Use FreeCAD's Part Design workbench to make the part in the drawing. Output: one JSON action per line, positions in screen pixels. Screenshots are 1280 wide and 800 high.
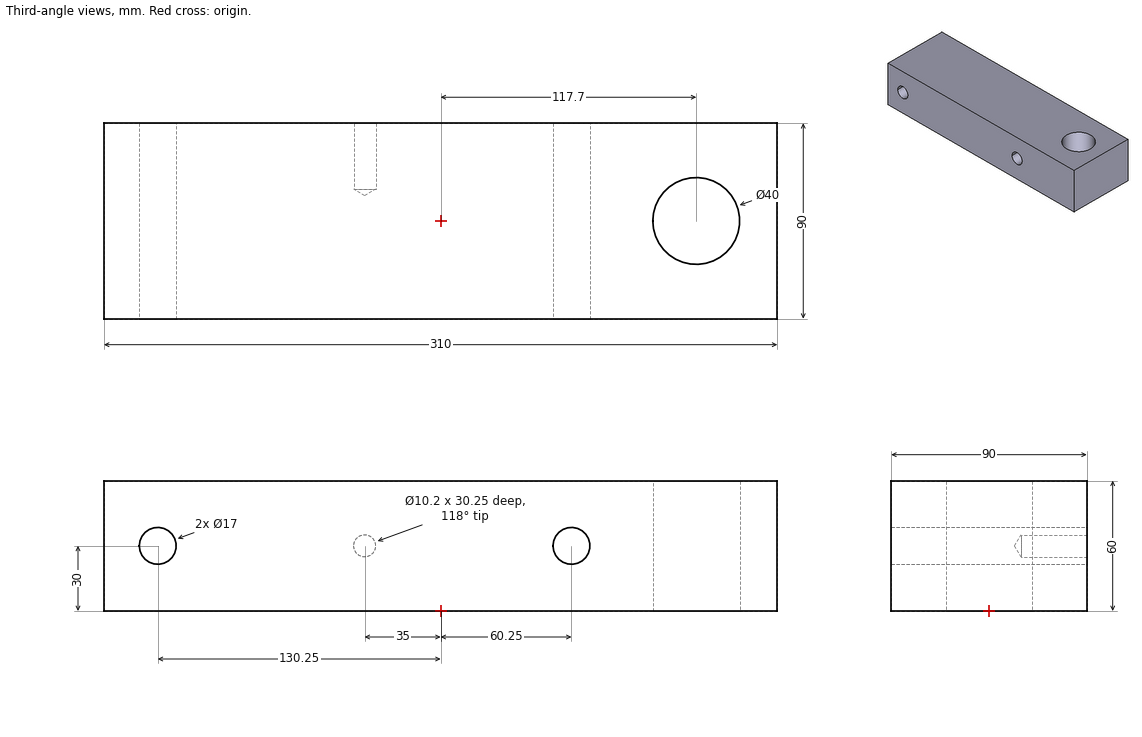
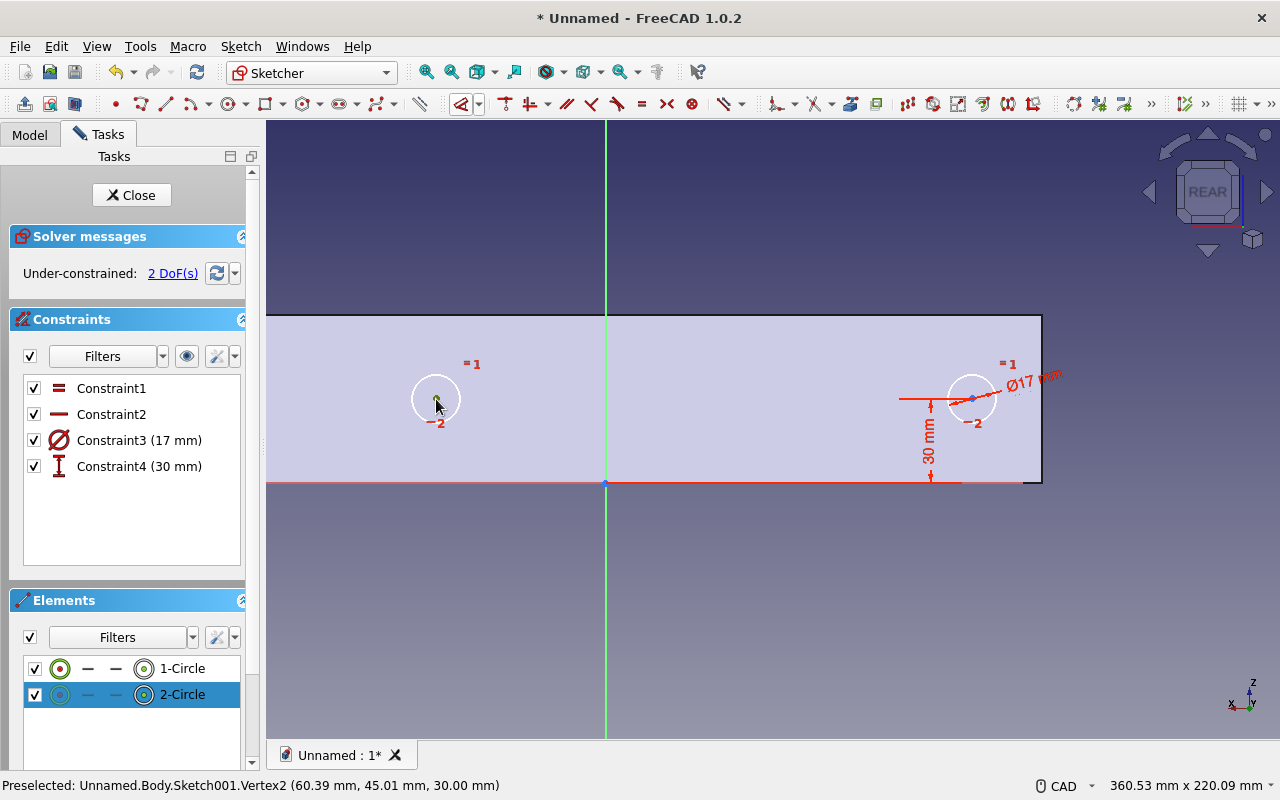
{"action": "key", "text": "l"}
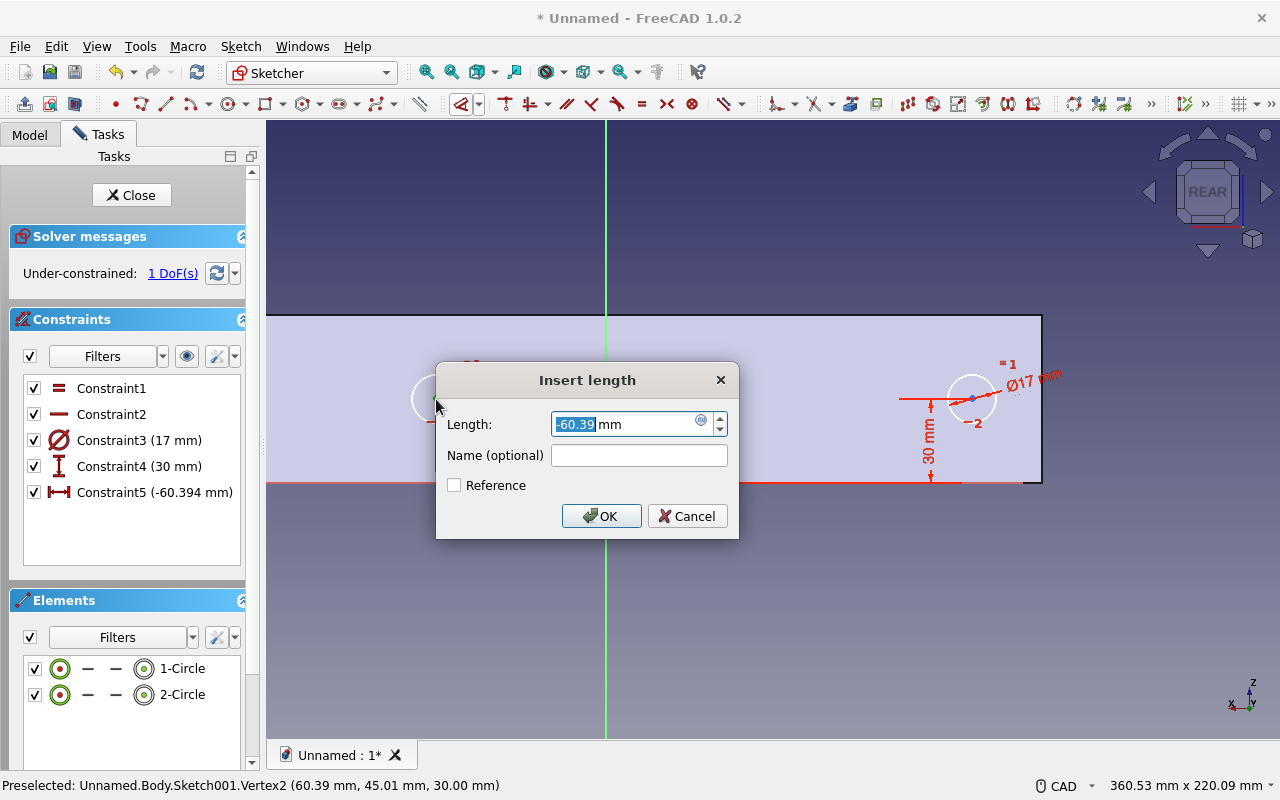
{"action": "type", "text": "-60.25"}
{"action": "key", "text": "Return"}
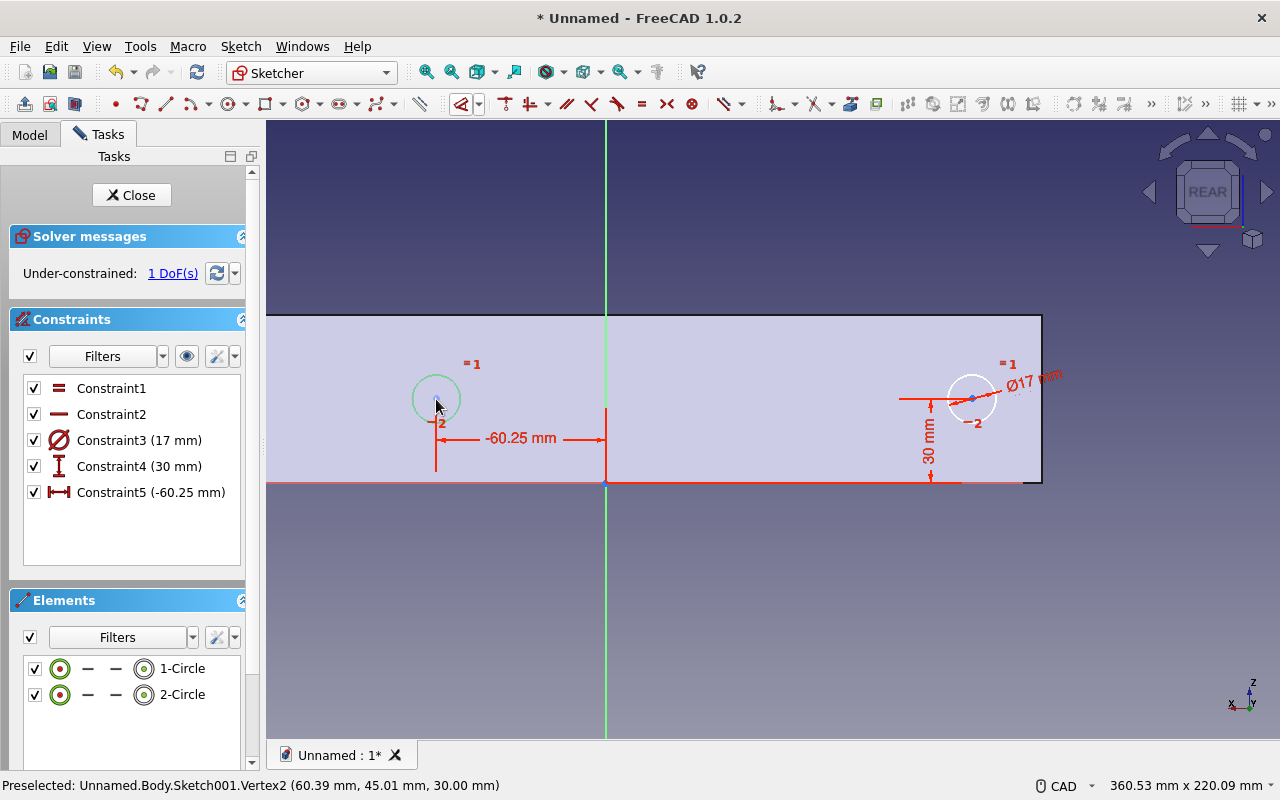
{"action": "left_click", "coordinate": [972, 399]}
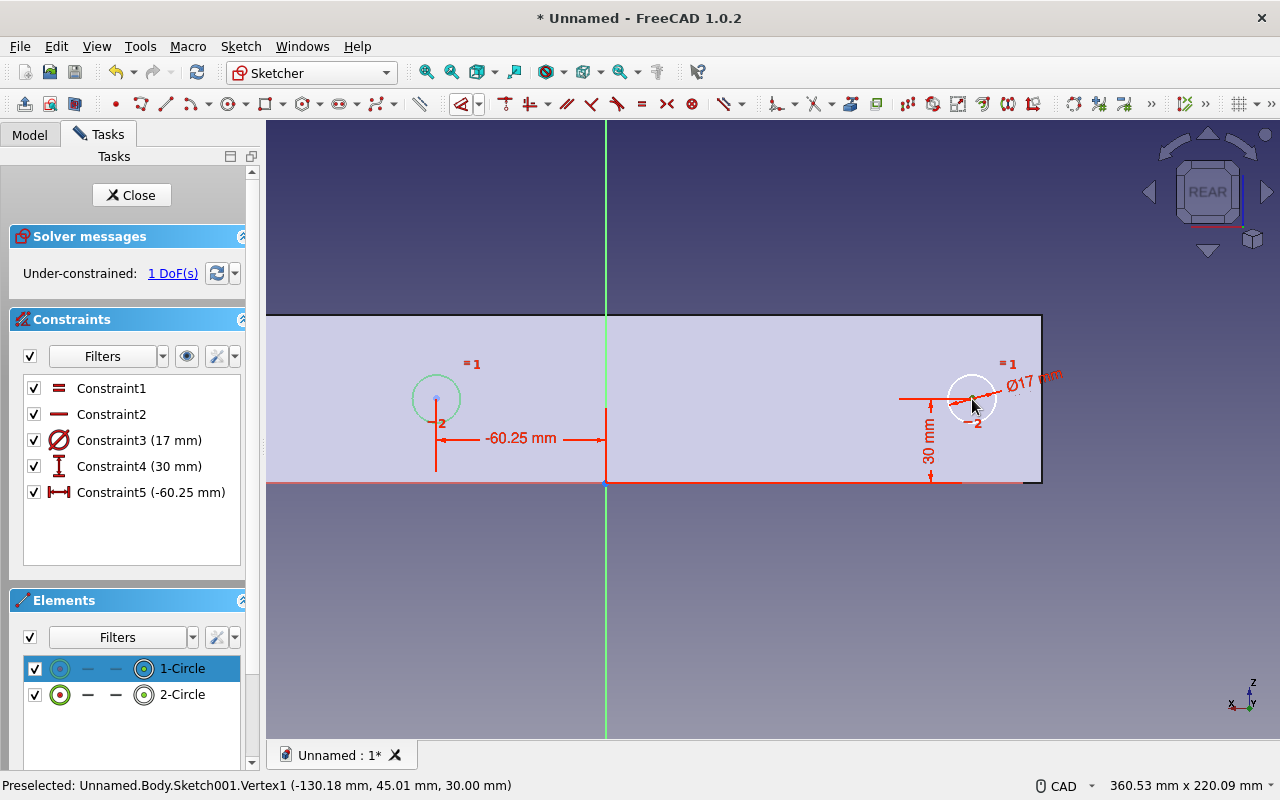
{"action": "left_click", "coordinate": [478, 104]}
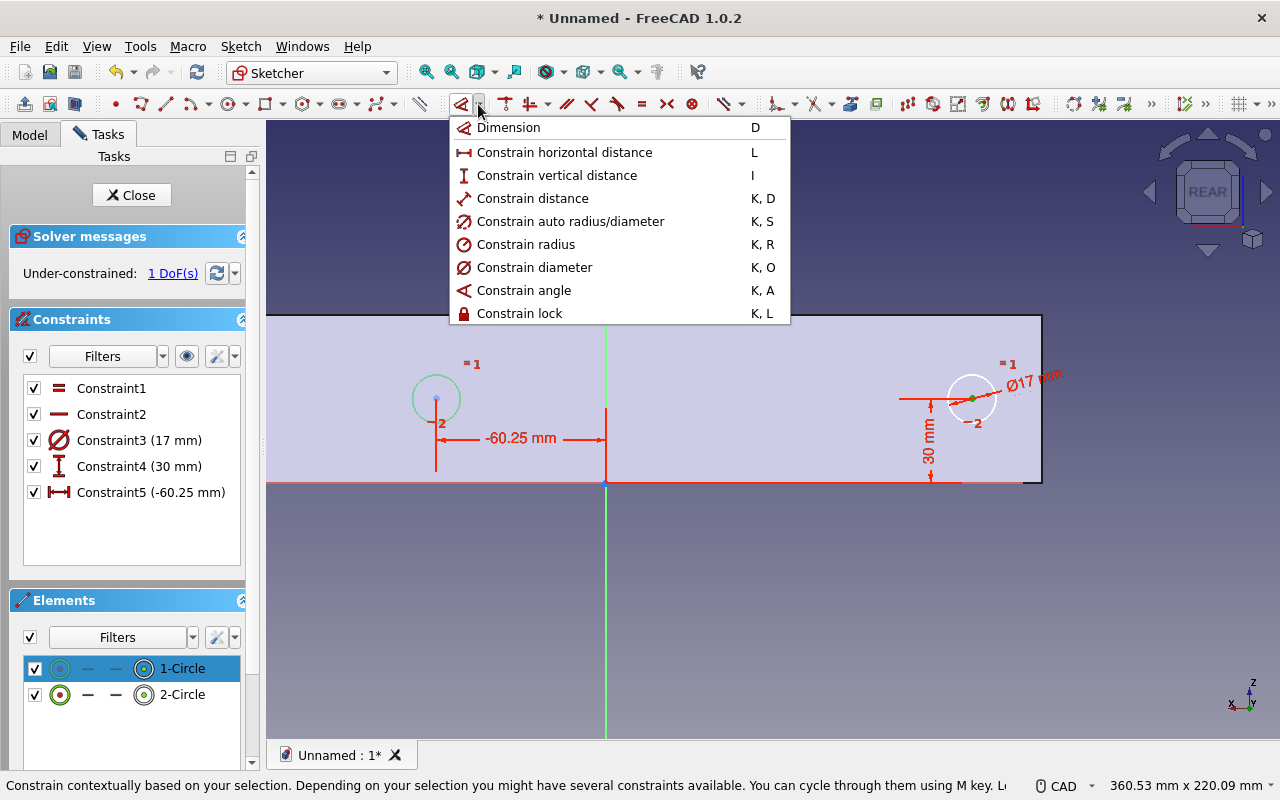
{"action": "left_click", "coordinate": [620, 152]}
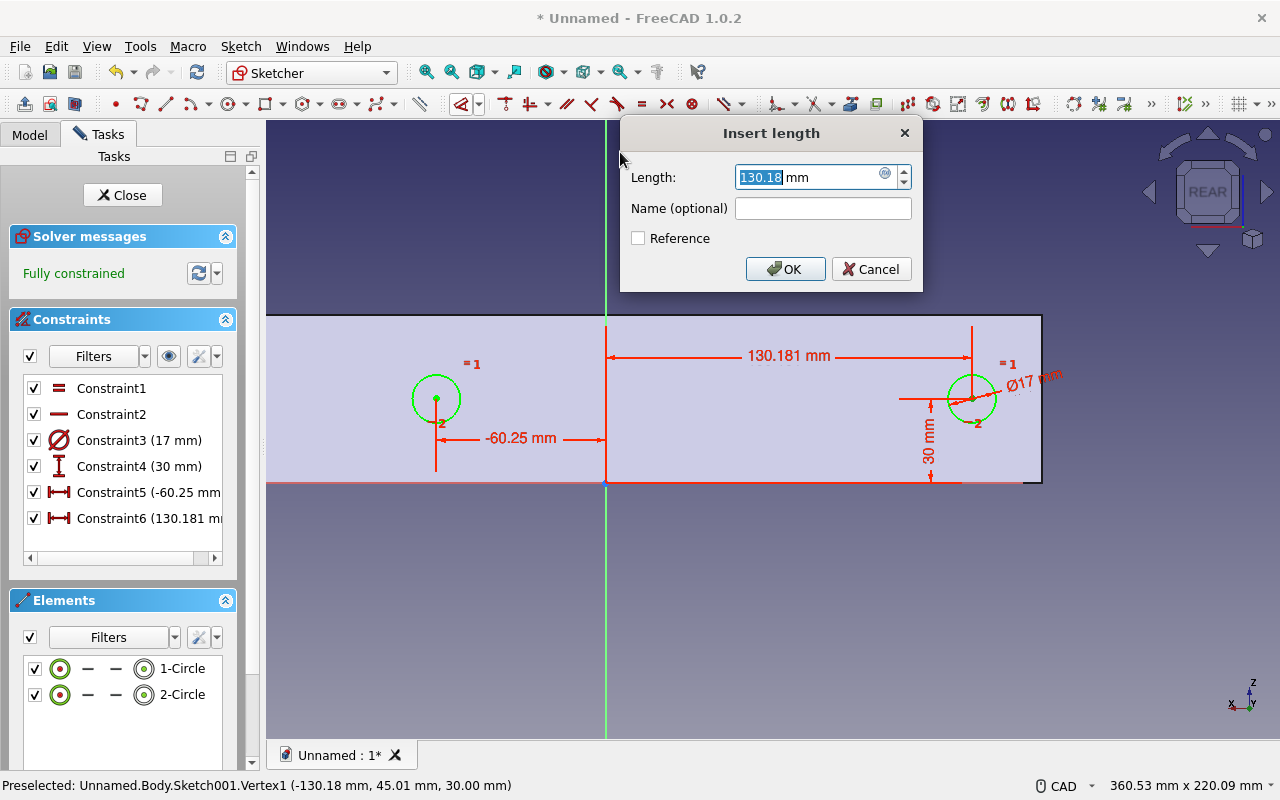
{"action": "type", "text": "130.25"}
{"action": "key", "text": "Return"}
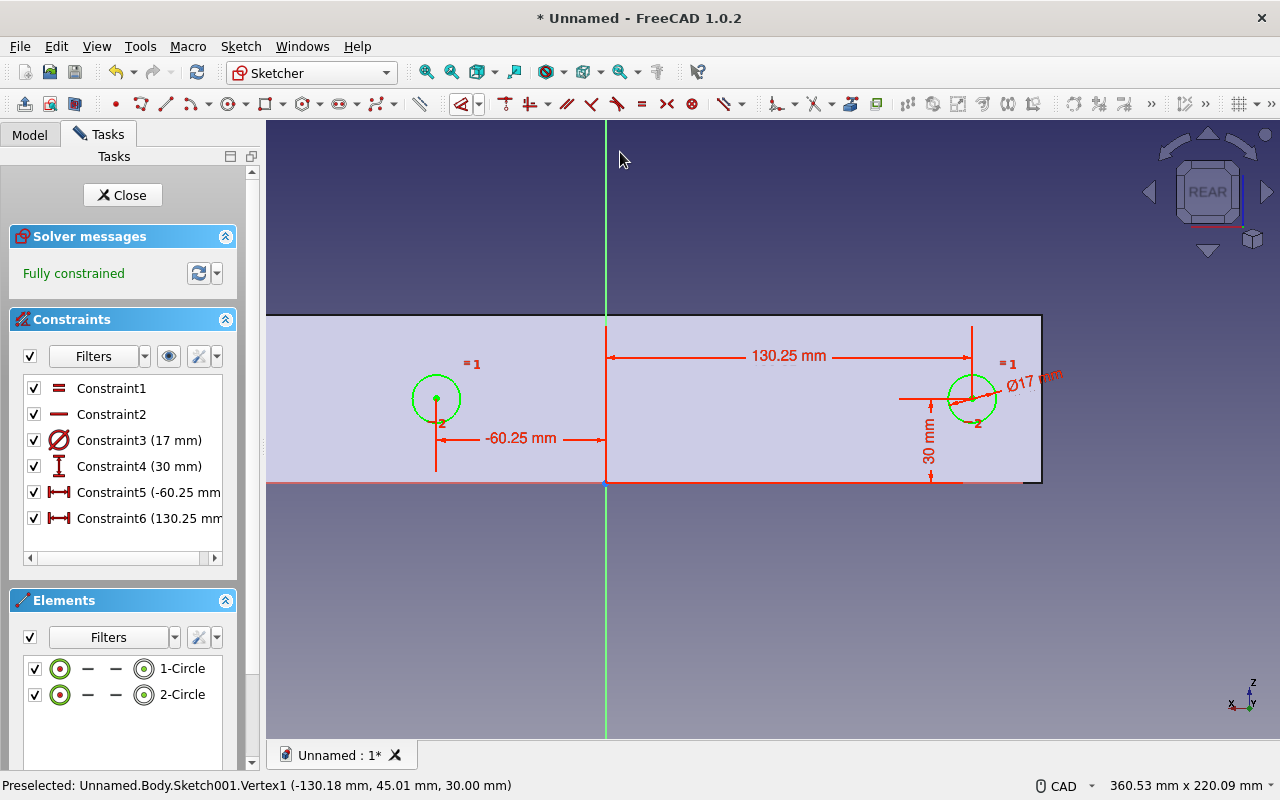
{"action": "left_click", "coordinate": [123, 195]}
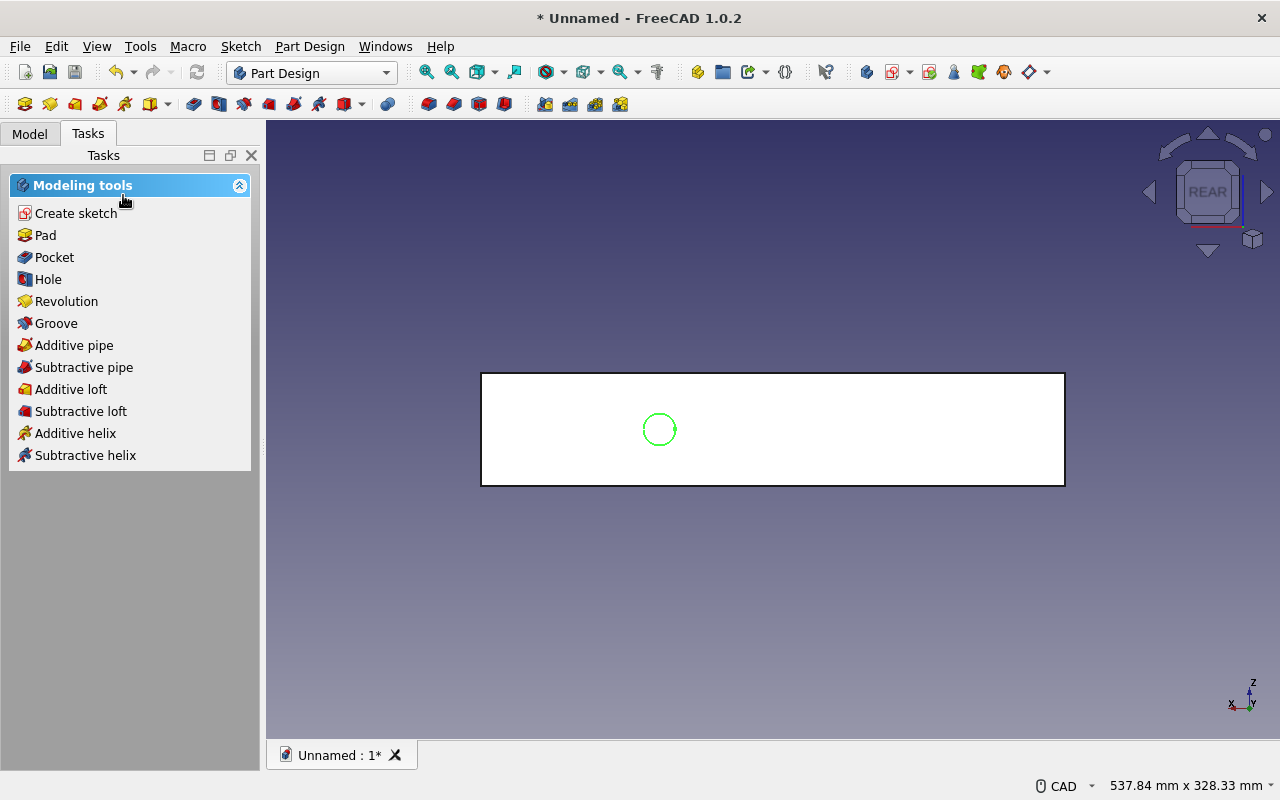
{"action": "left_click", "coordinate": [194, 104]}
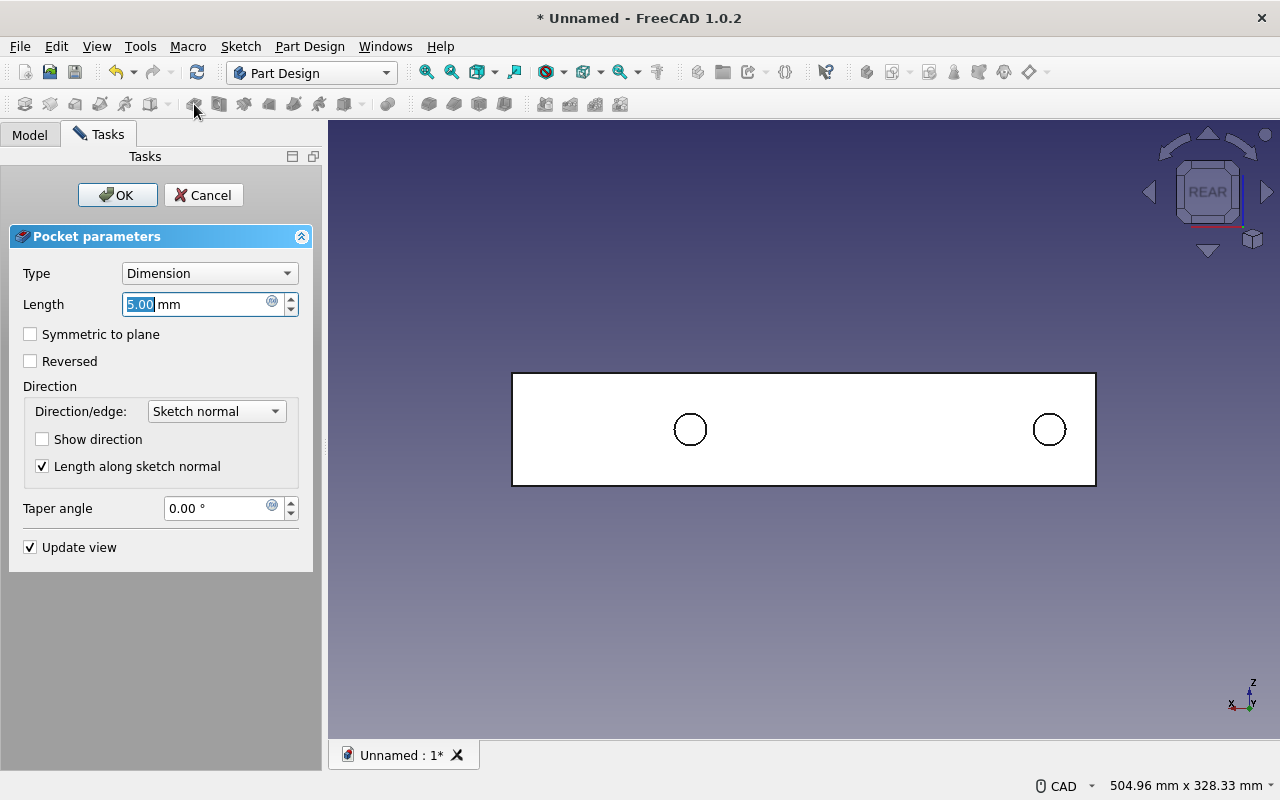
{"action": "type", "text": "90"}
{"action": "key", "text": "Tab"}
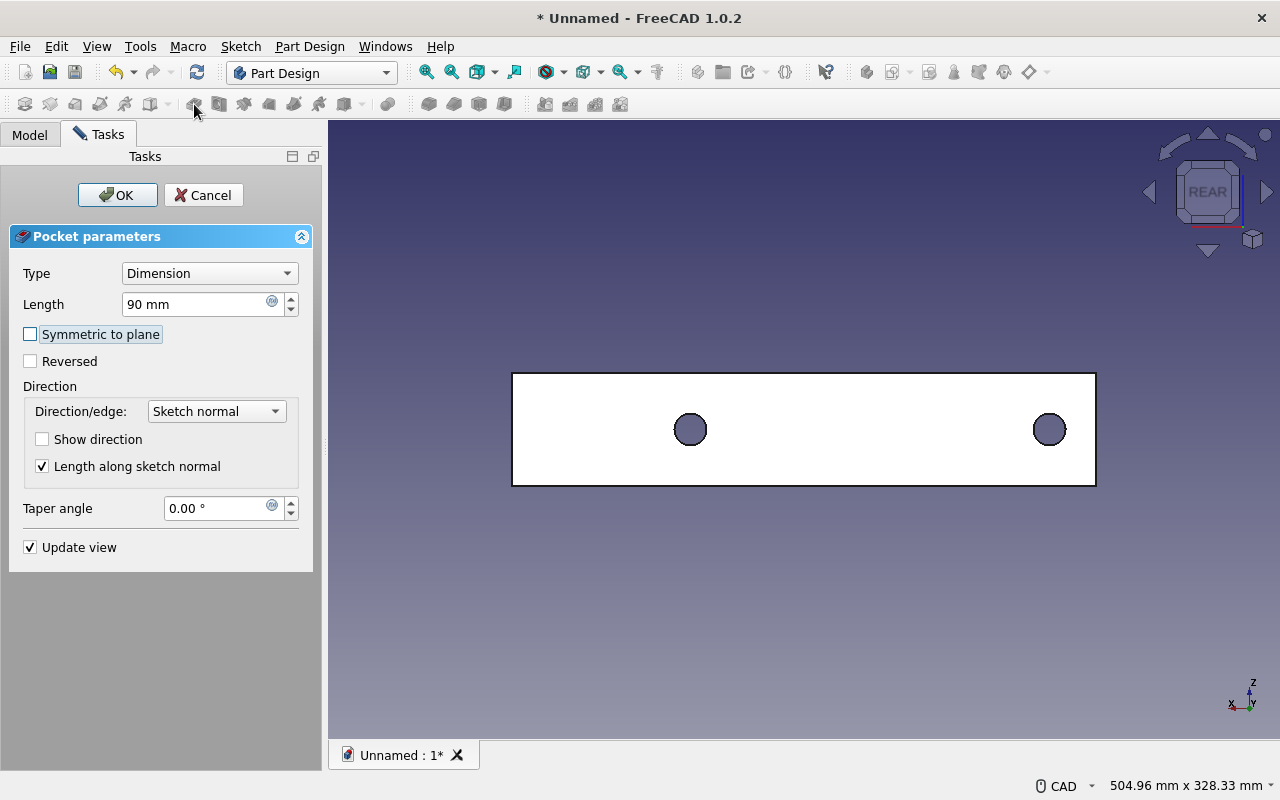
{"action": "left_click", "coordinate": [118, 195]}